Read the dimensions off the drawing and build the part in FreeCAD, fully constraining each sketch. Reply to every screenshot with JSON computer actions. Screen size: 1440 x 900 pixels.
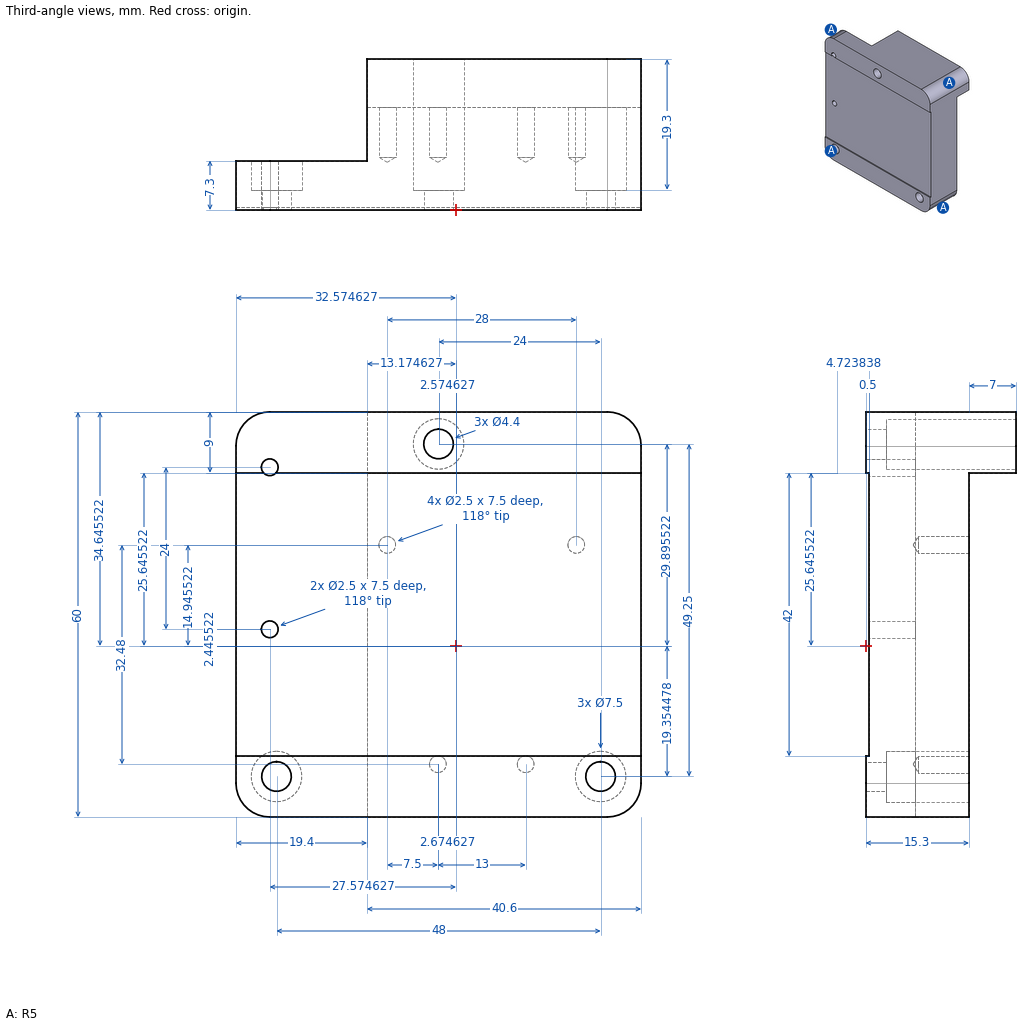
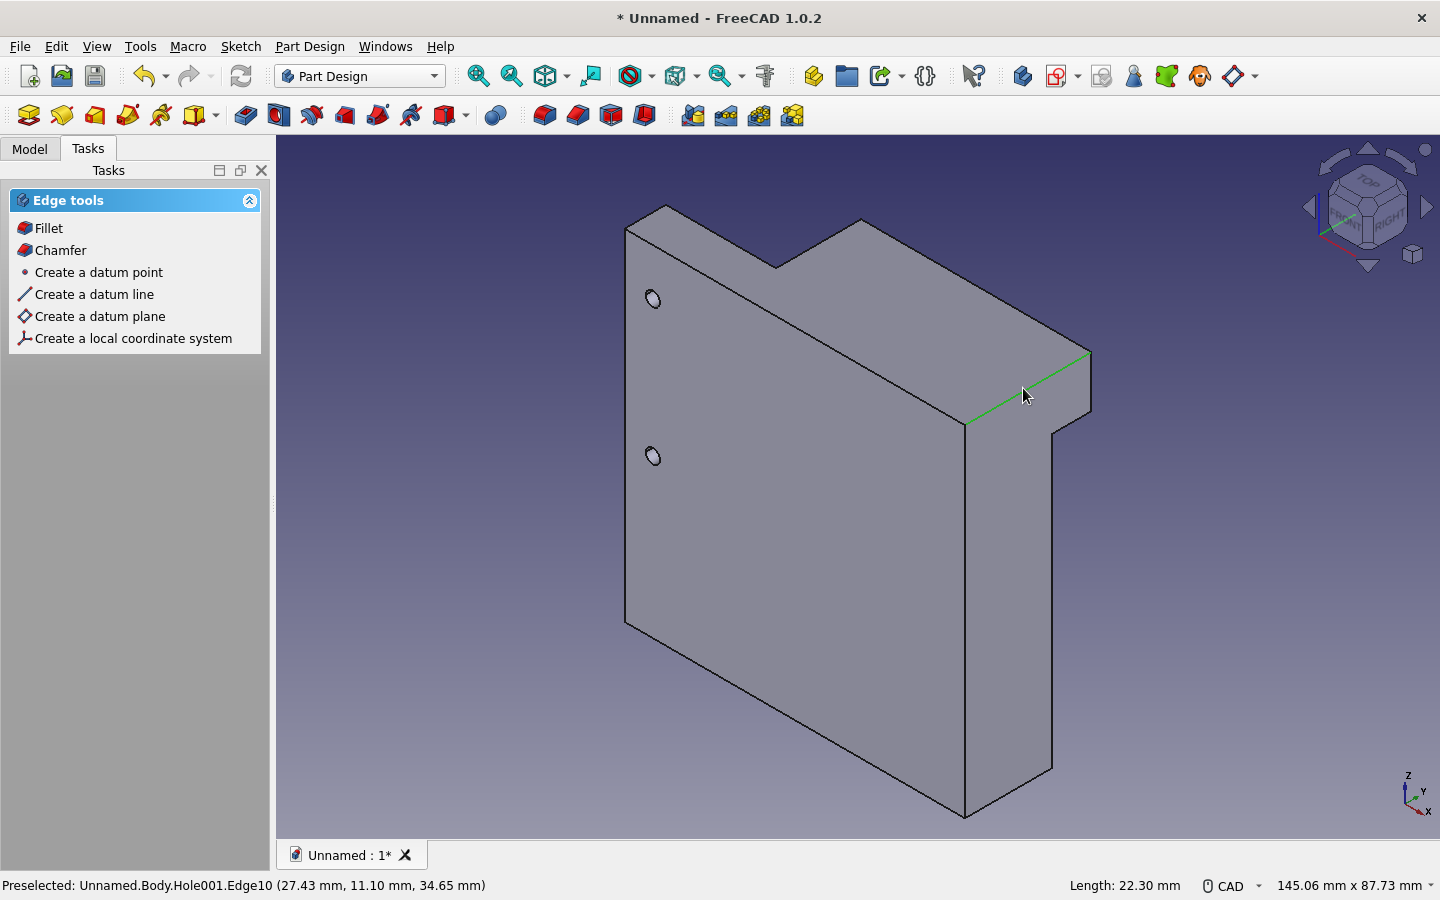
{"action": "key", "text": "2"}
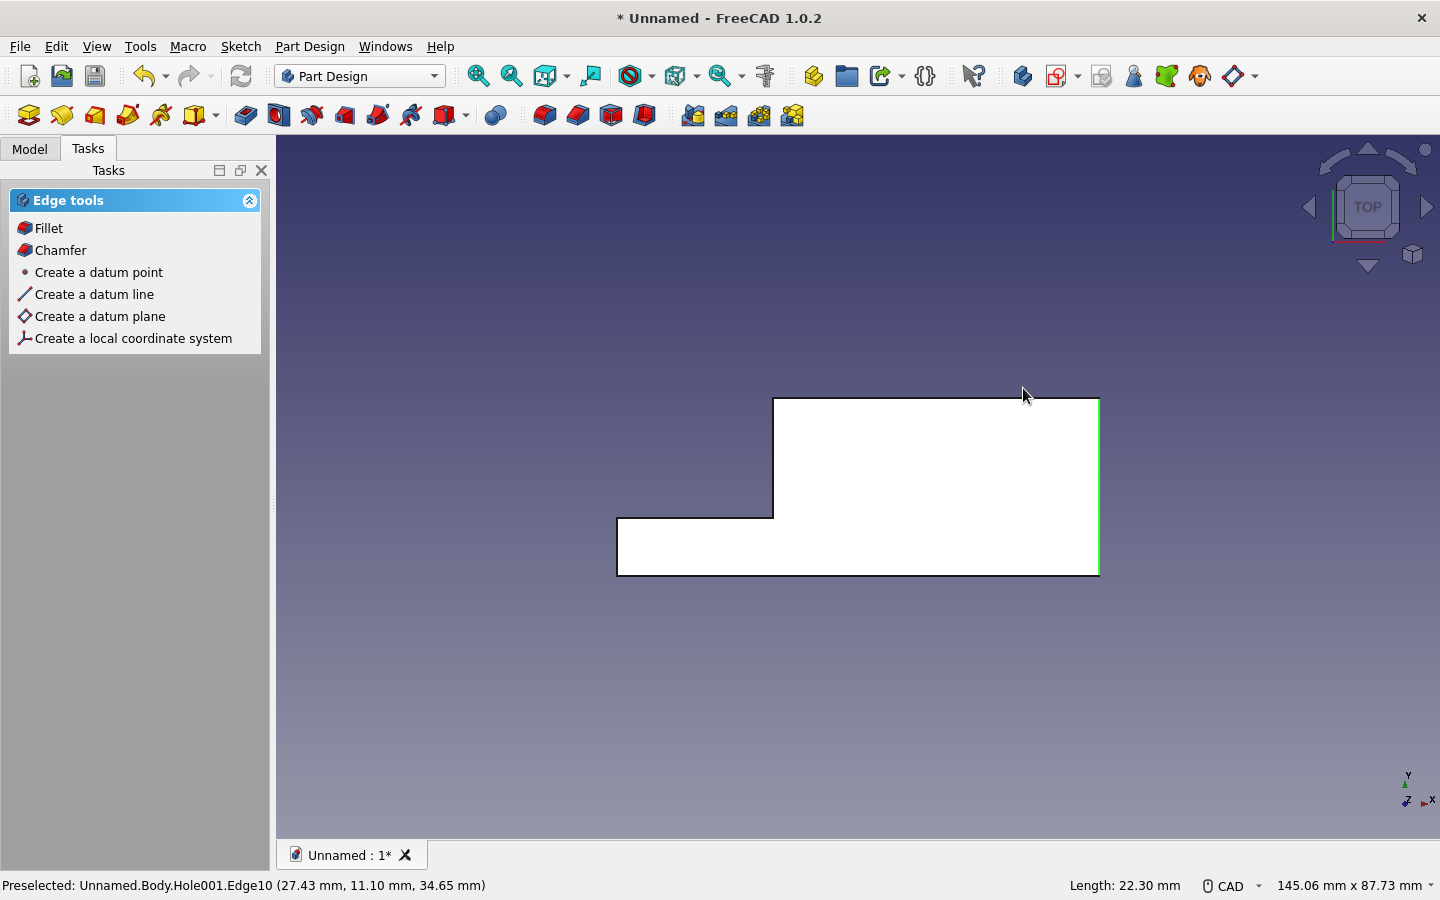
{"action": "key", "text": "v f"}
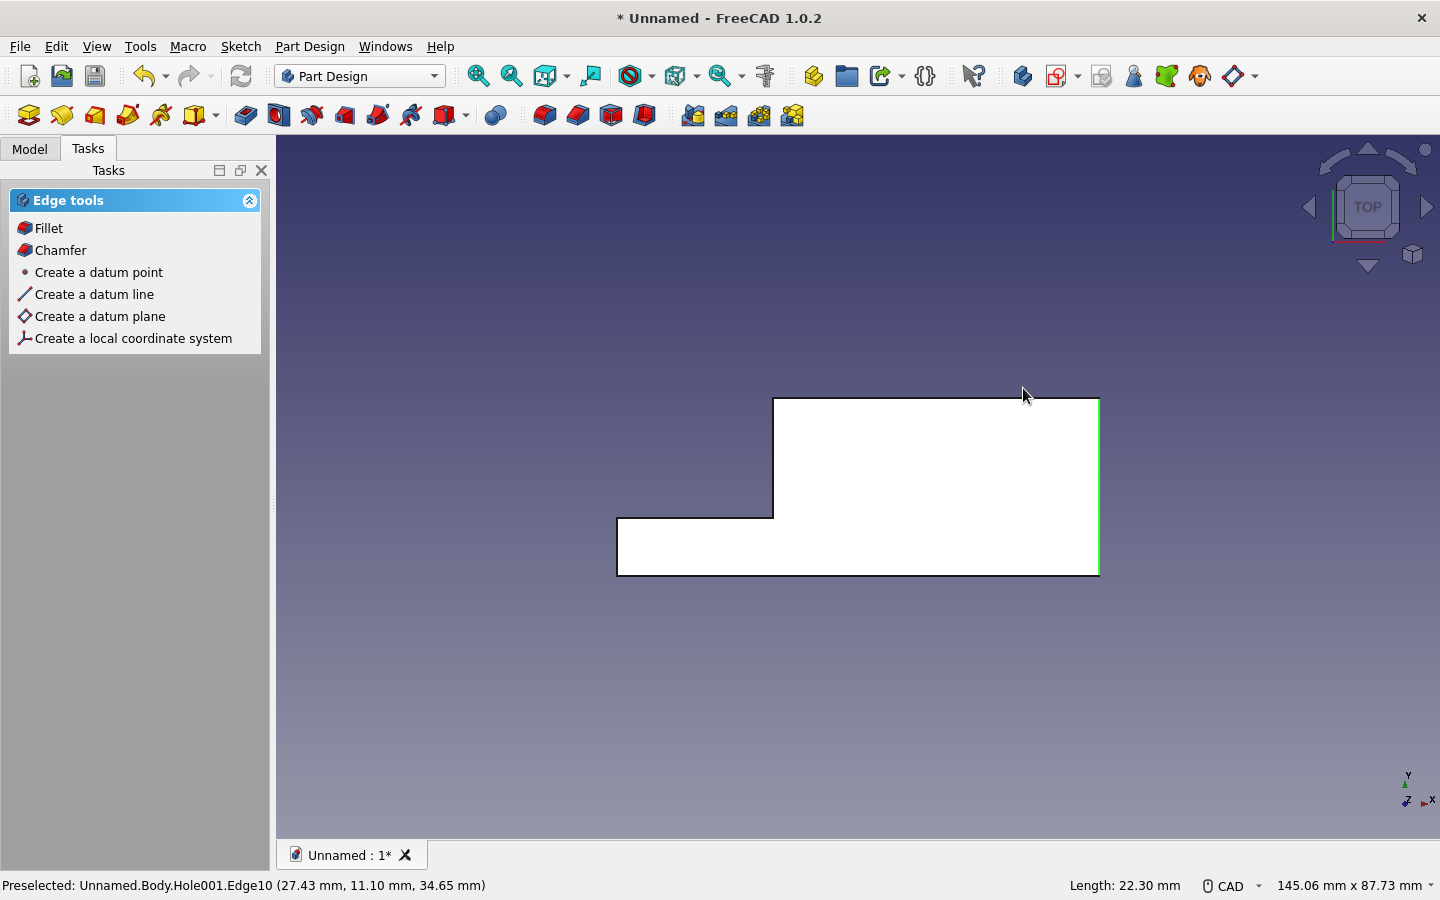
{"action": "left_click", "coordinate": [617, 546], "text": "ctrl"}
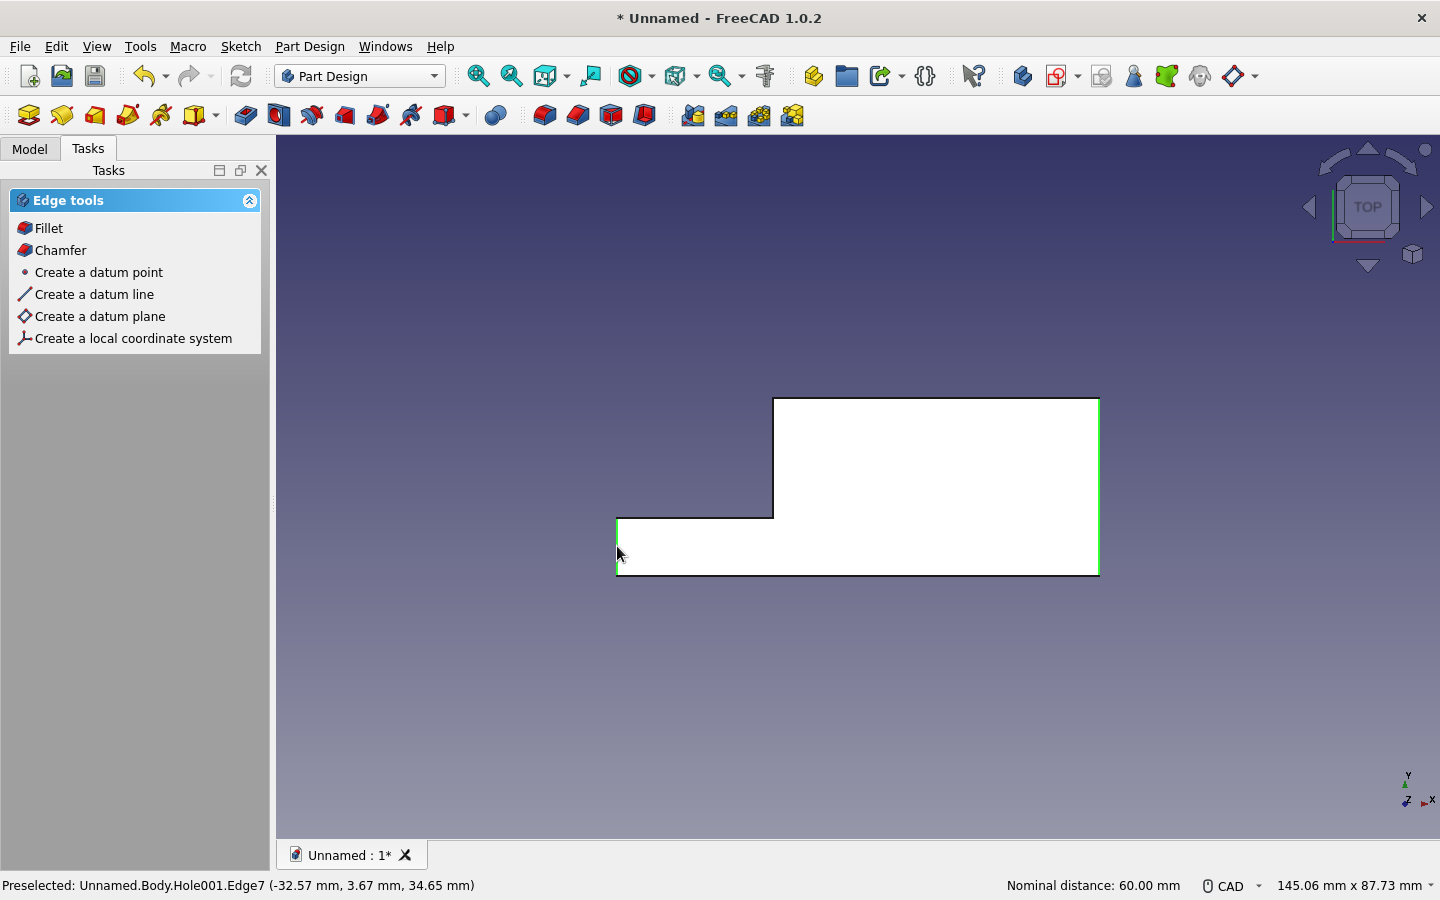
{"action": "key", "text": "1"}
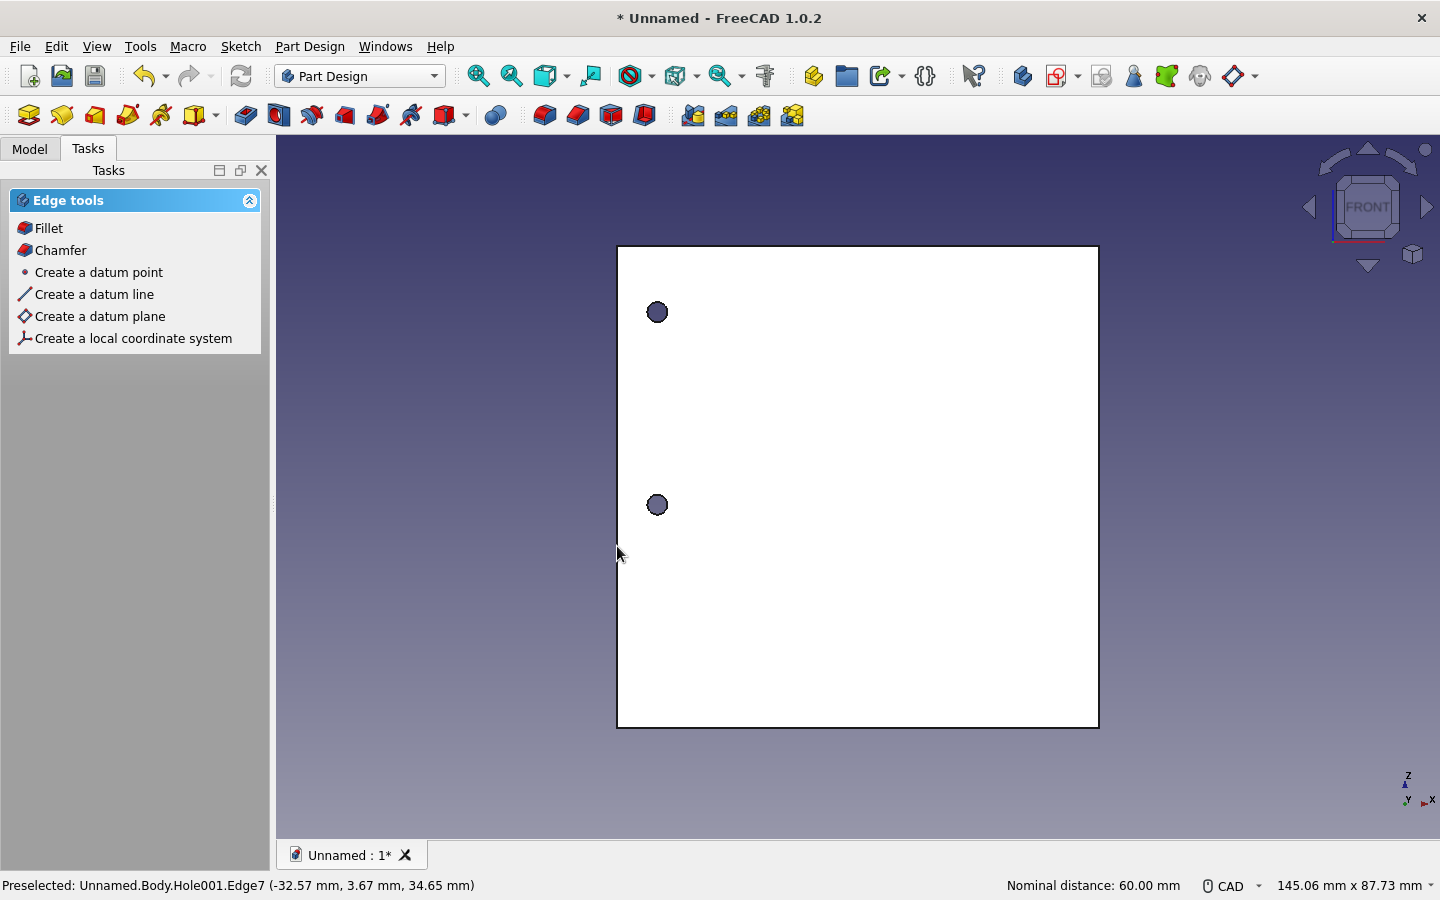
{"action": "key", "text": "3"}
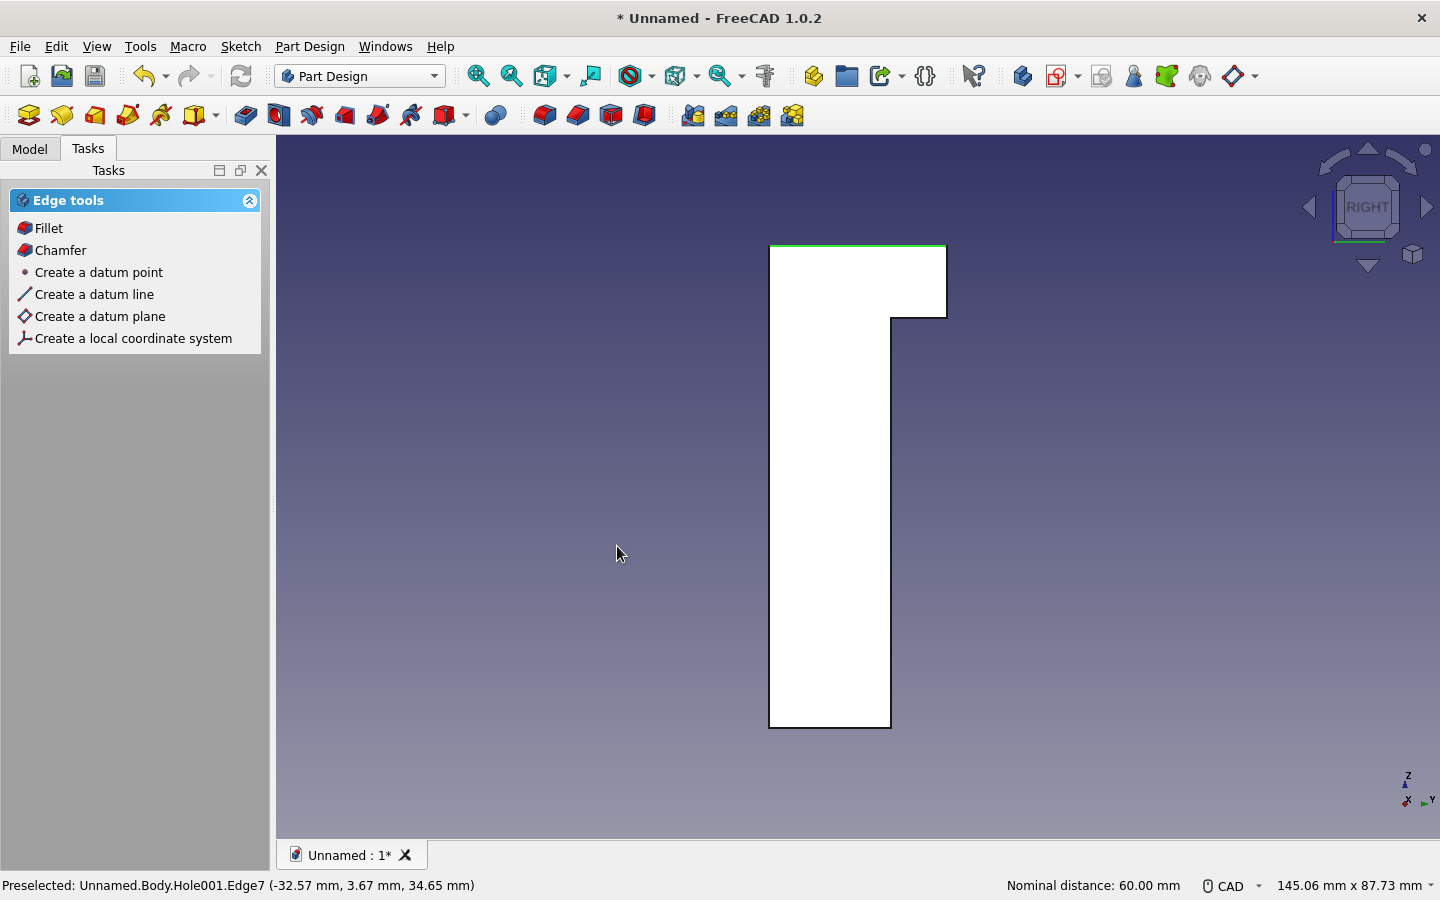
{"action": "left_click", "coordinate": [830, 727], "text": "ctrl"}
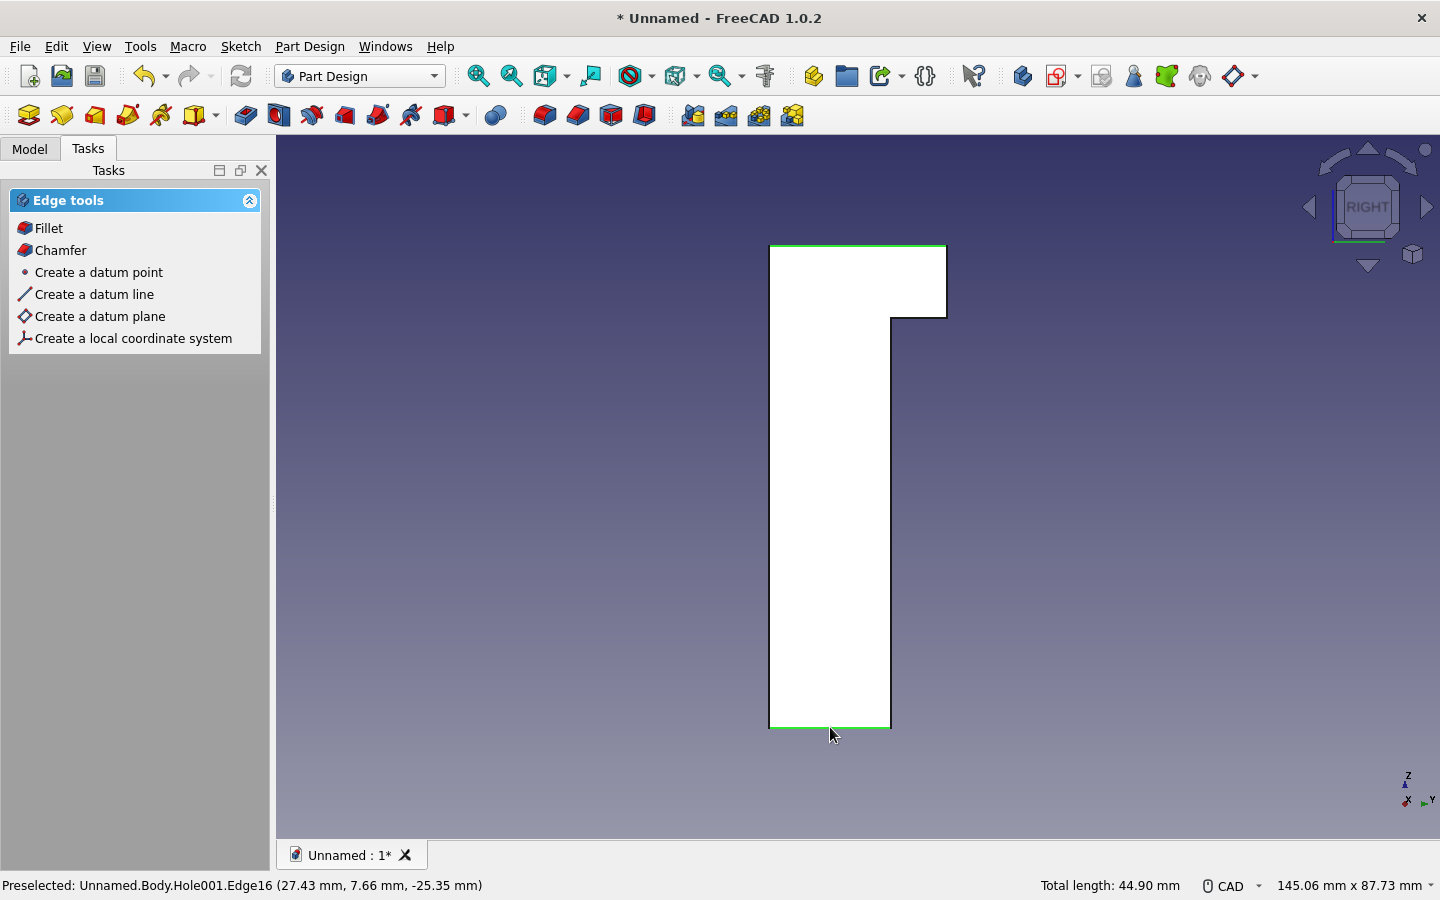
{"action": "key", "text": "5"}